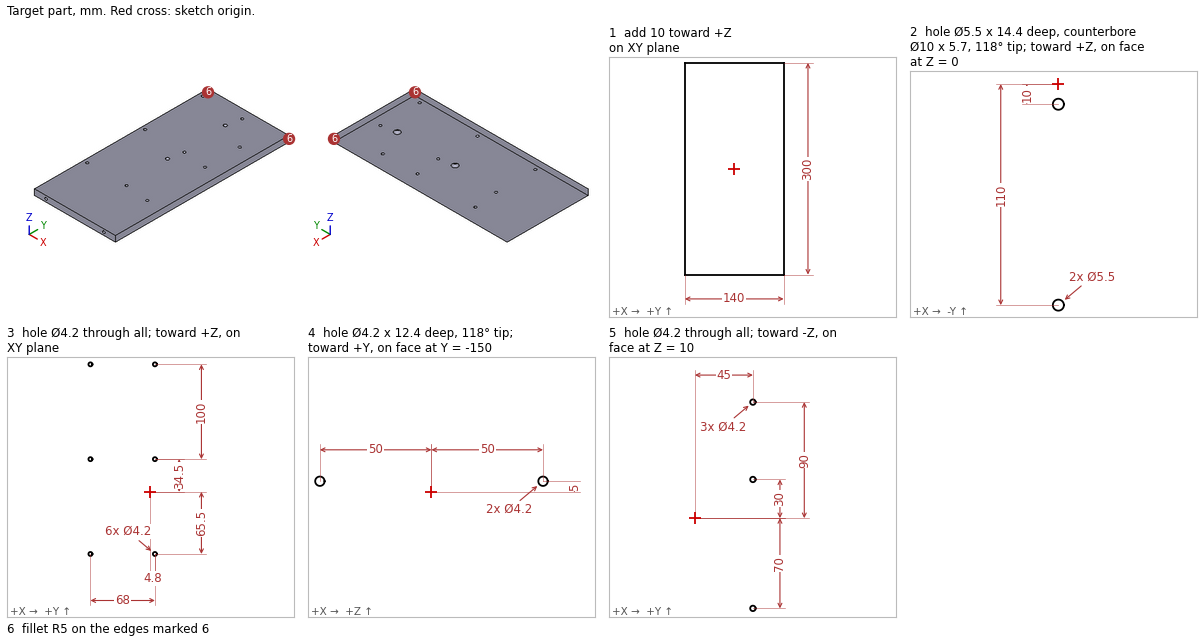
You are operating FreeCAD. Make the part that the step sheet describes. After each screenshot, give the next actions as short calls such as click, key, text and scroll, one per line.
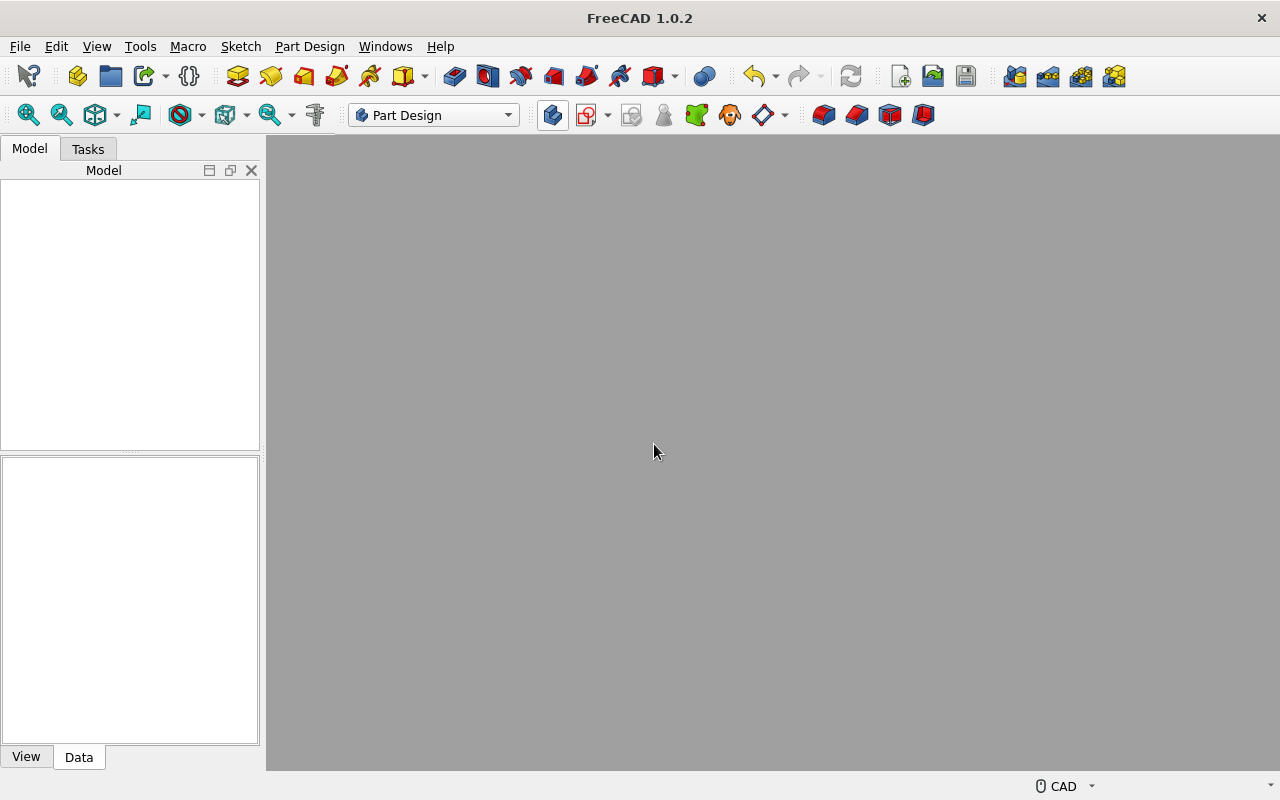
click(900, 76)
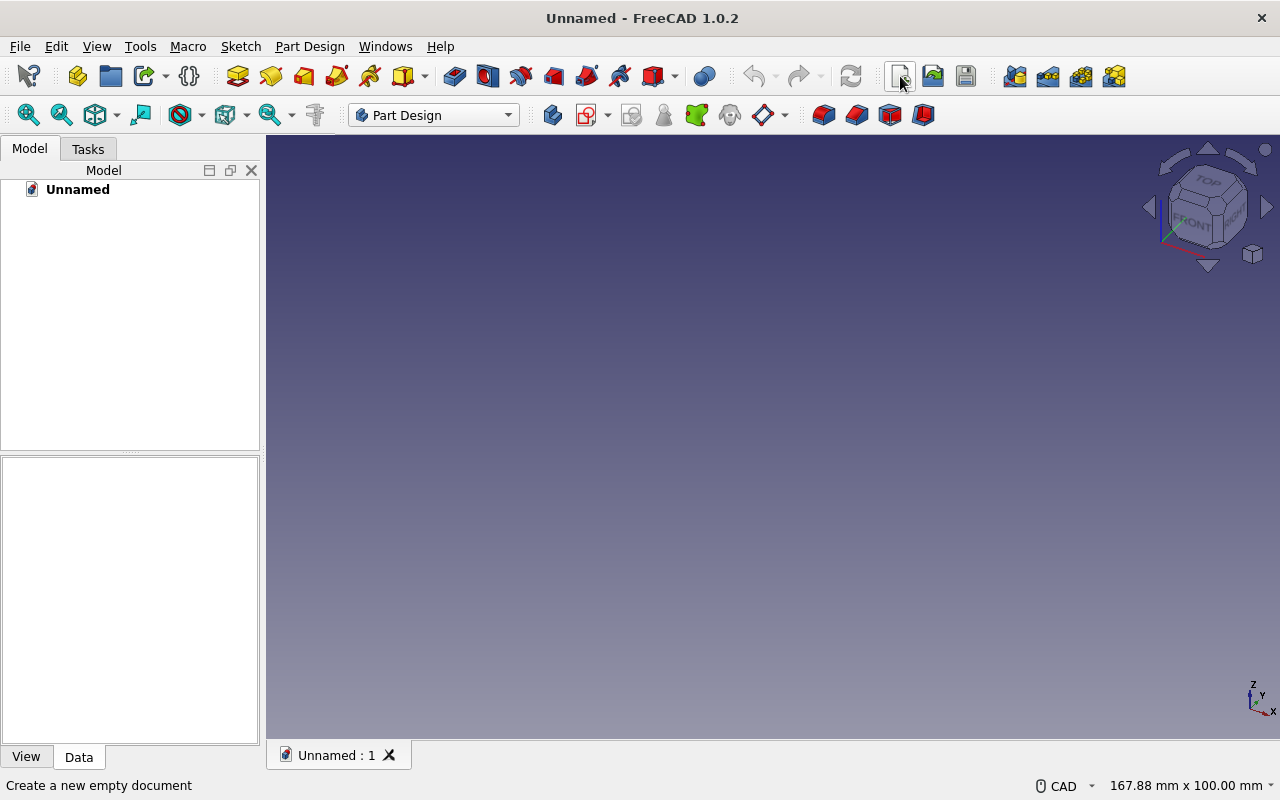
click(586, 116)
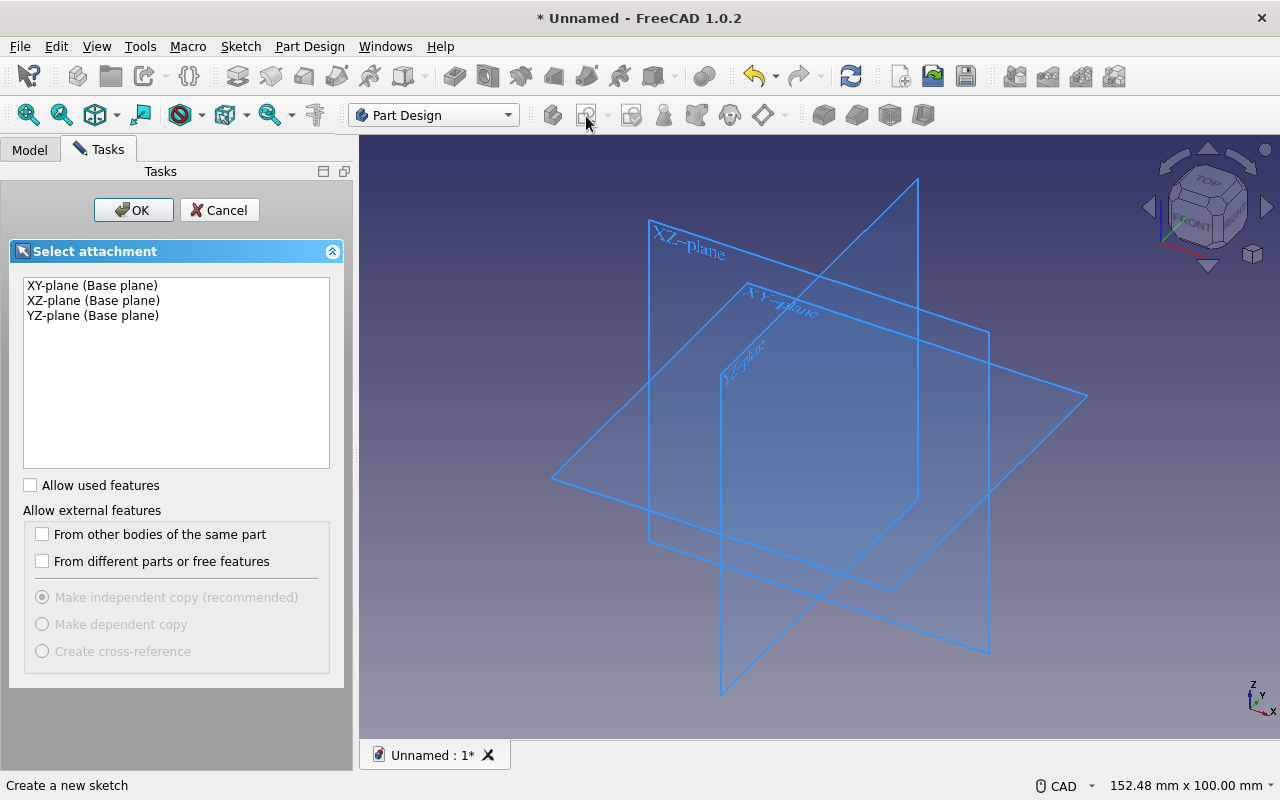
click(84, 286)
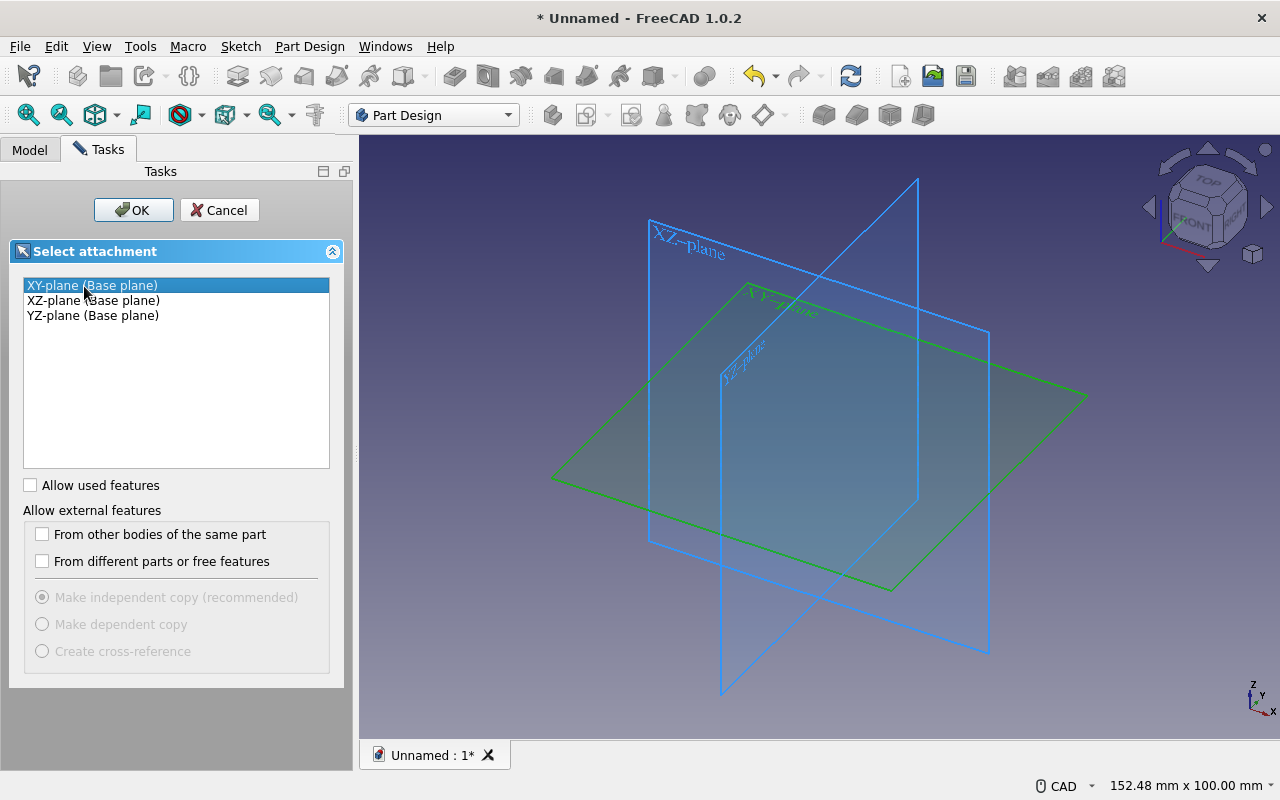
click(134, 210)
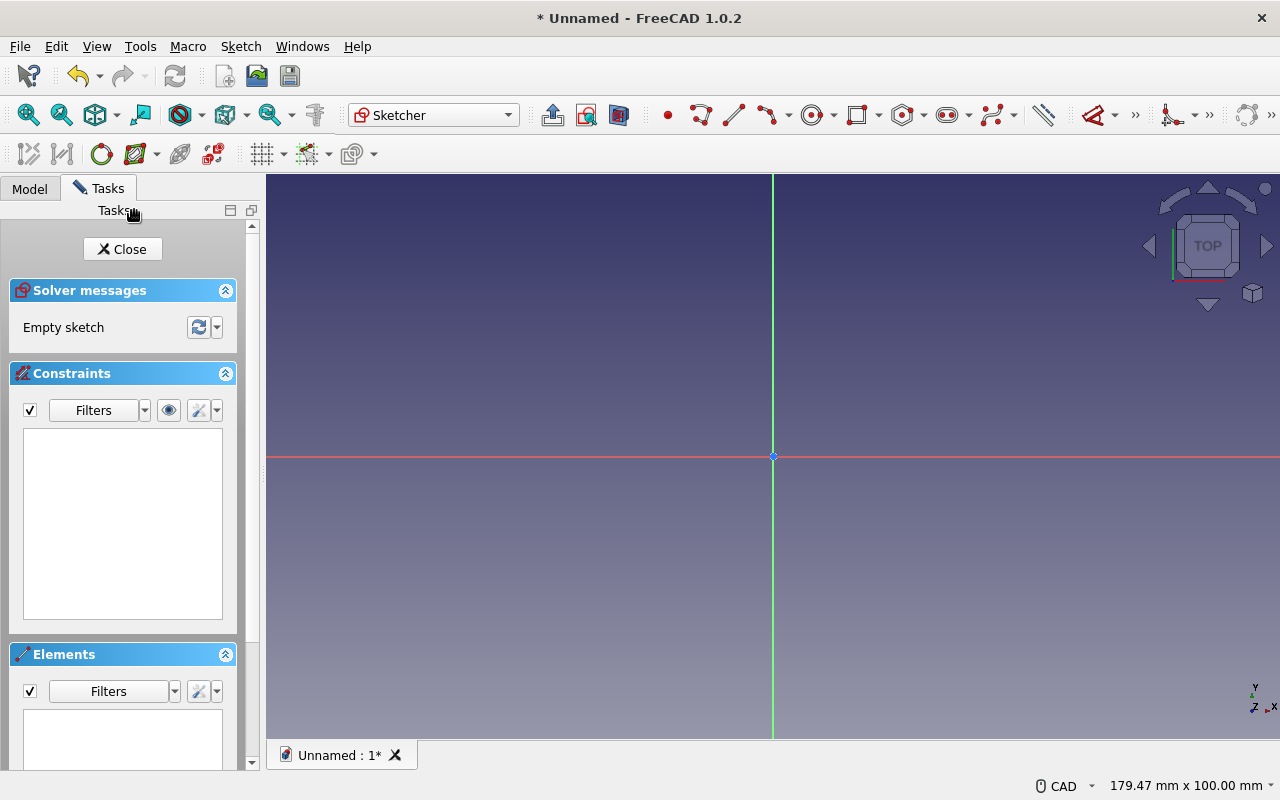
scroll(687, 456, down, 8)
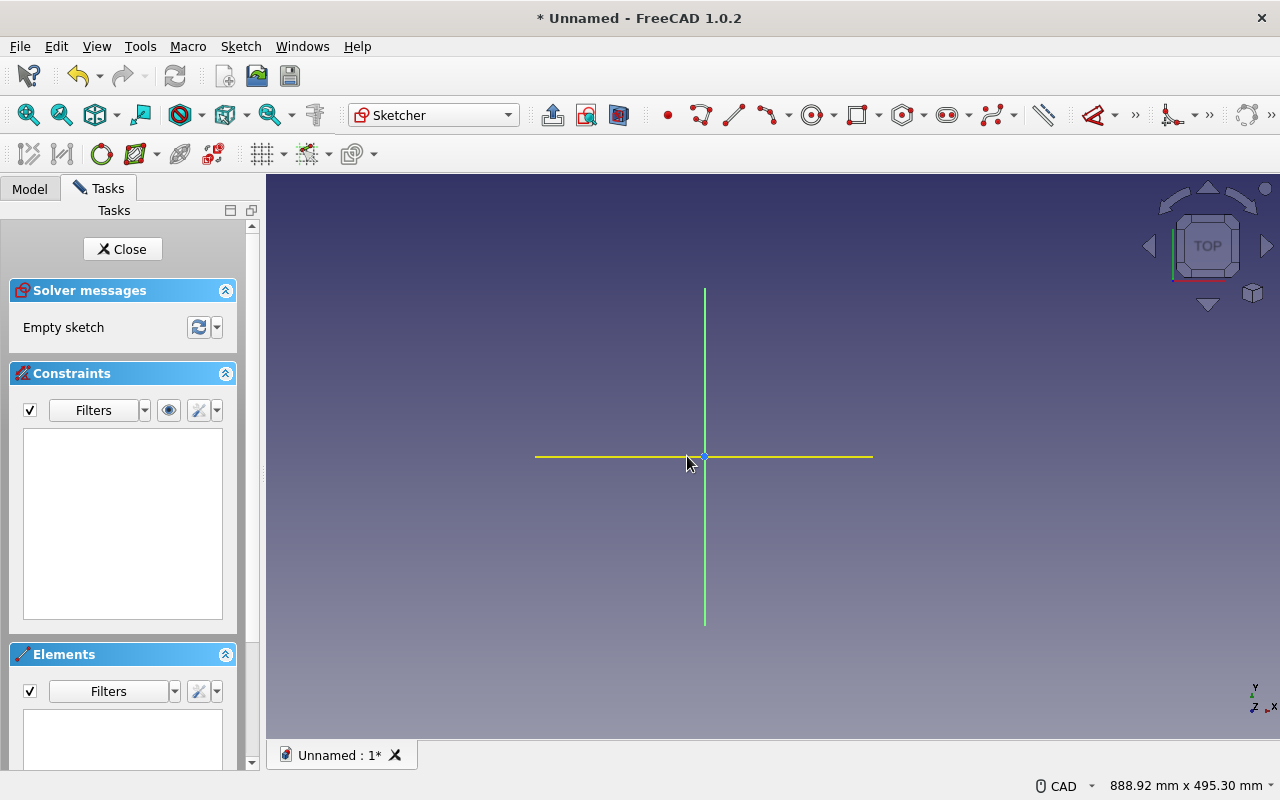
click(878, 116)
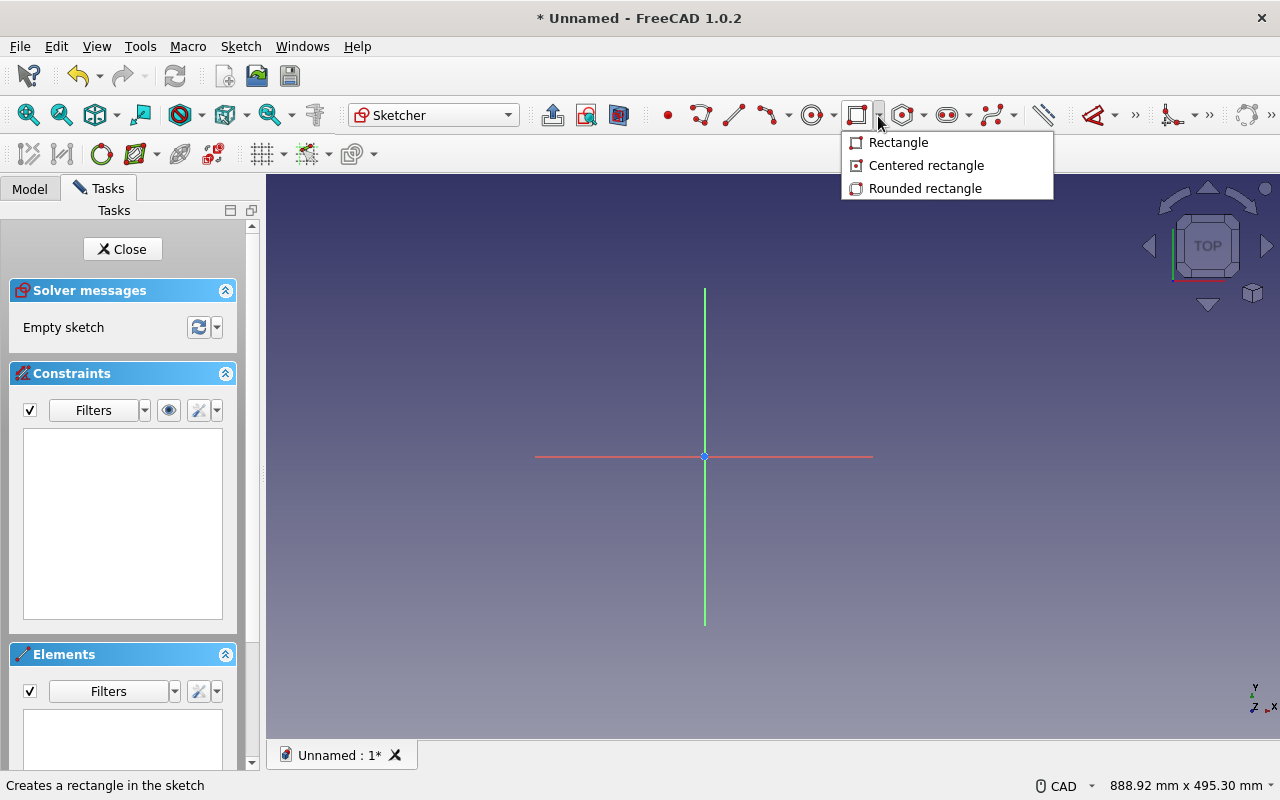
click(948, 166)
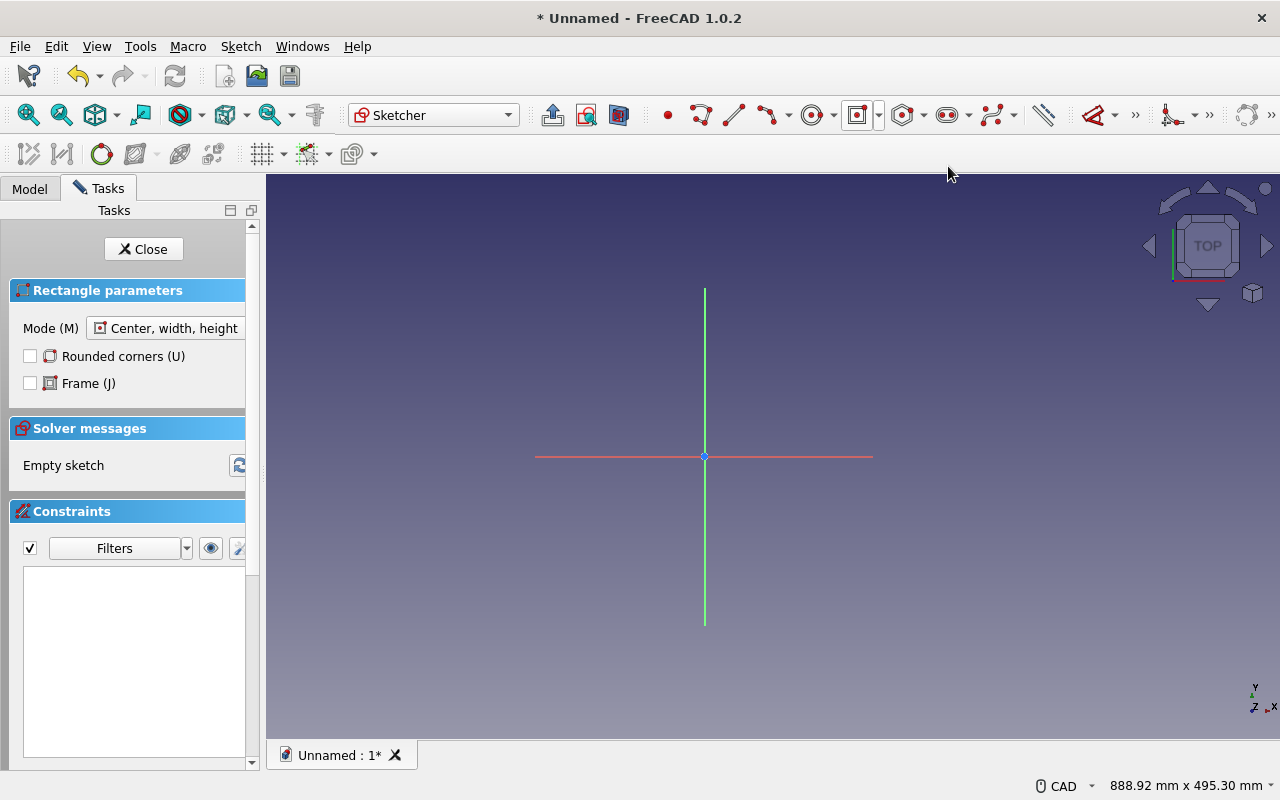
click(705, 456)
click(785, 285)
key(Escape)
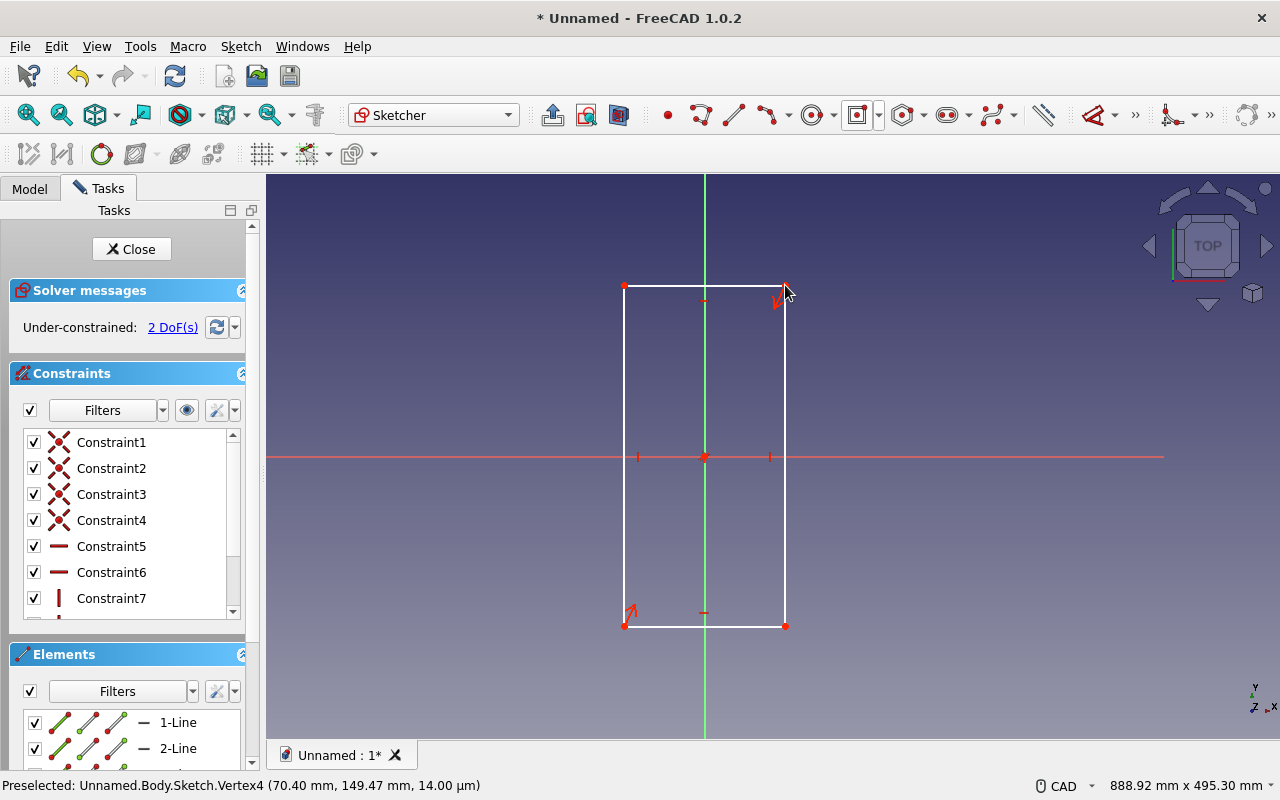
click(1092, 116)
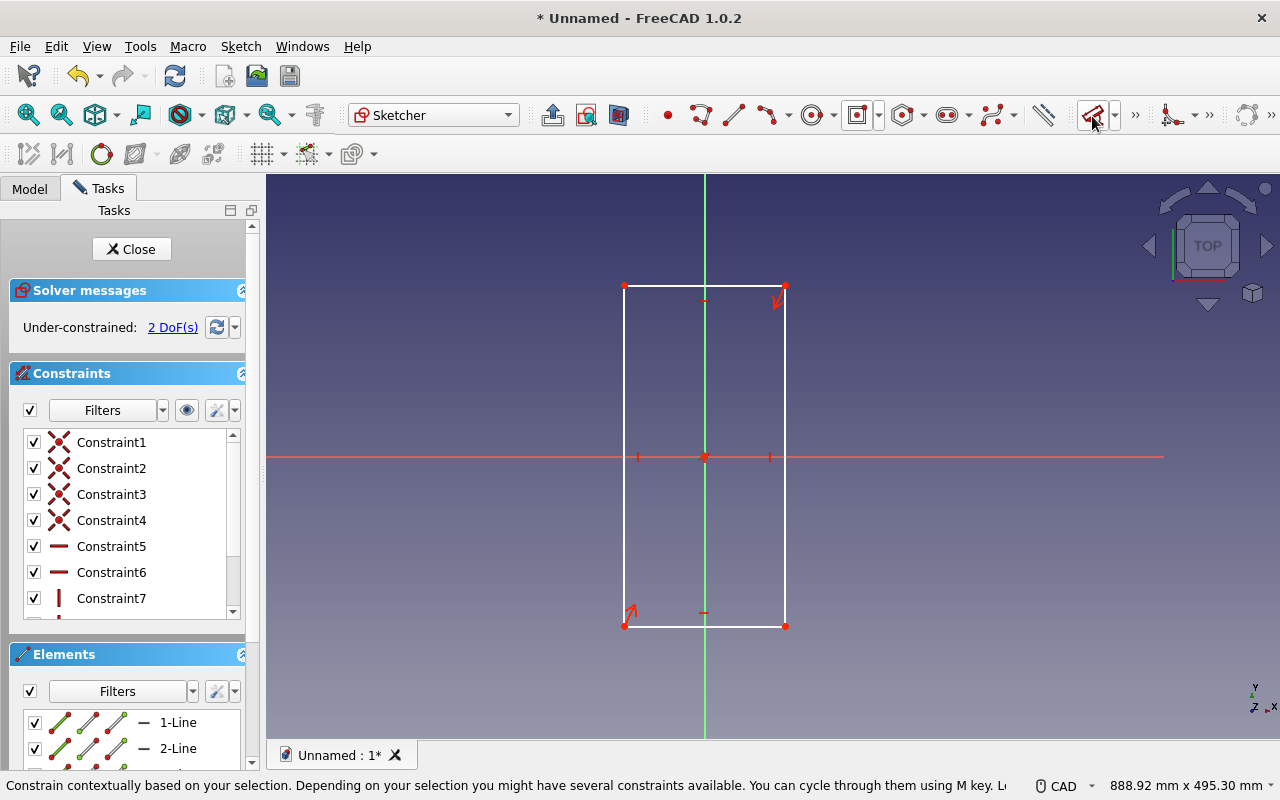
click(673, 627)
click(668, 661)